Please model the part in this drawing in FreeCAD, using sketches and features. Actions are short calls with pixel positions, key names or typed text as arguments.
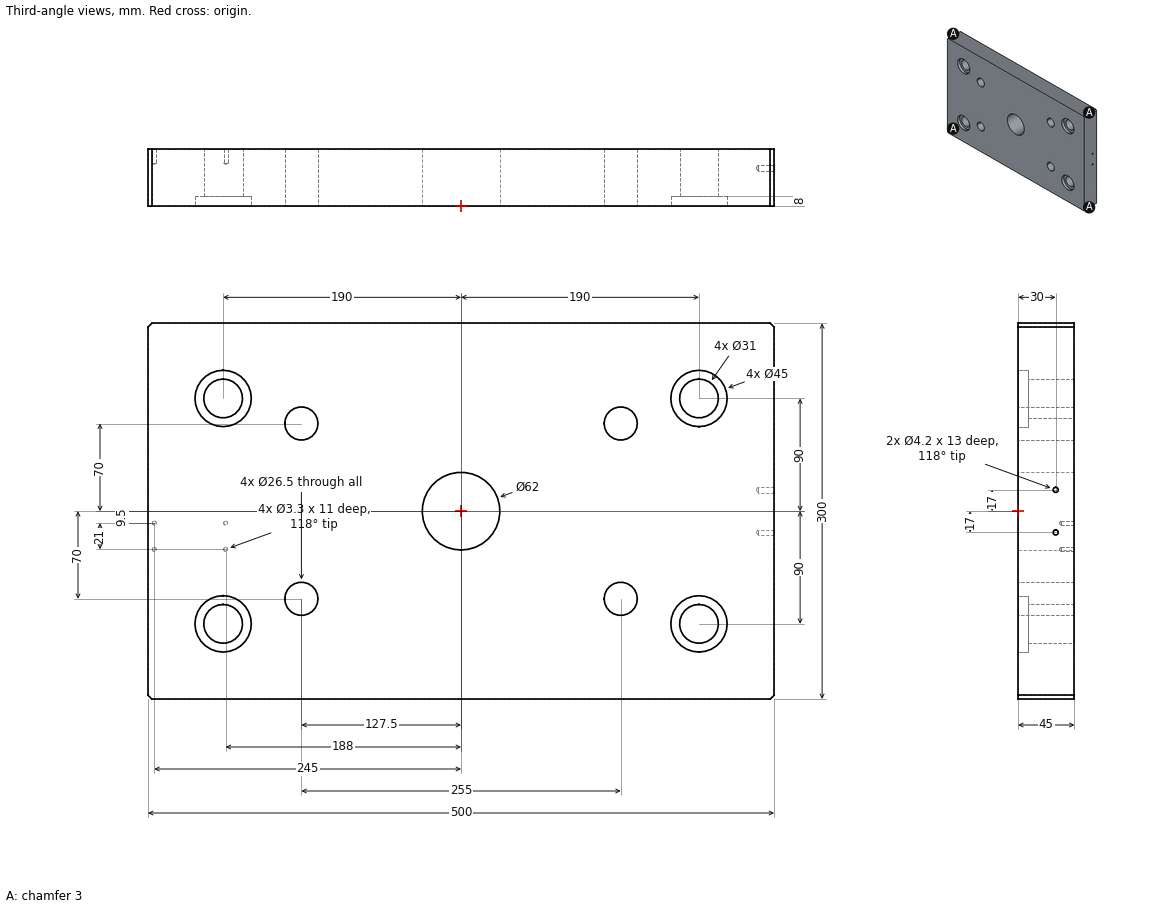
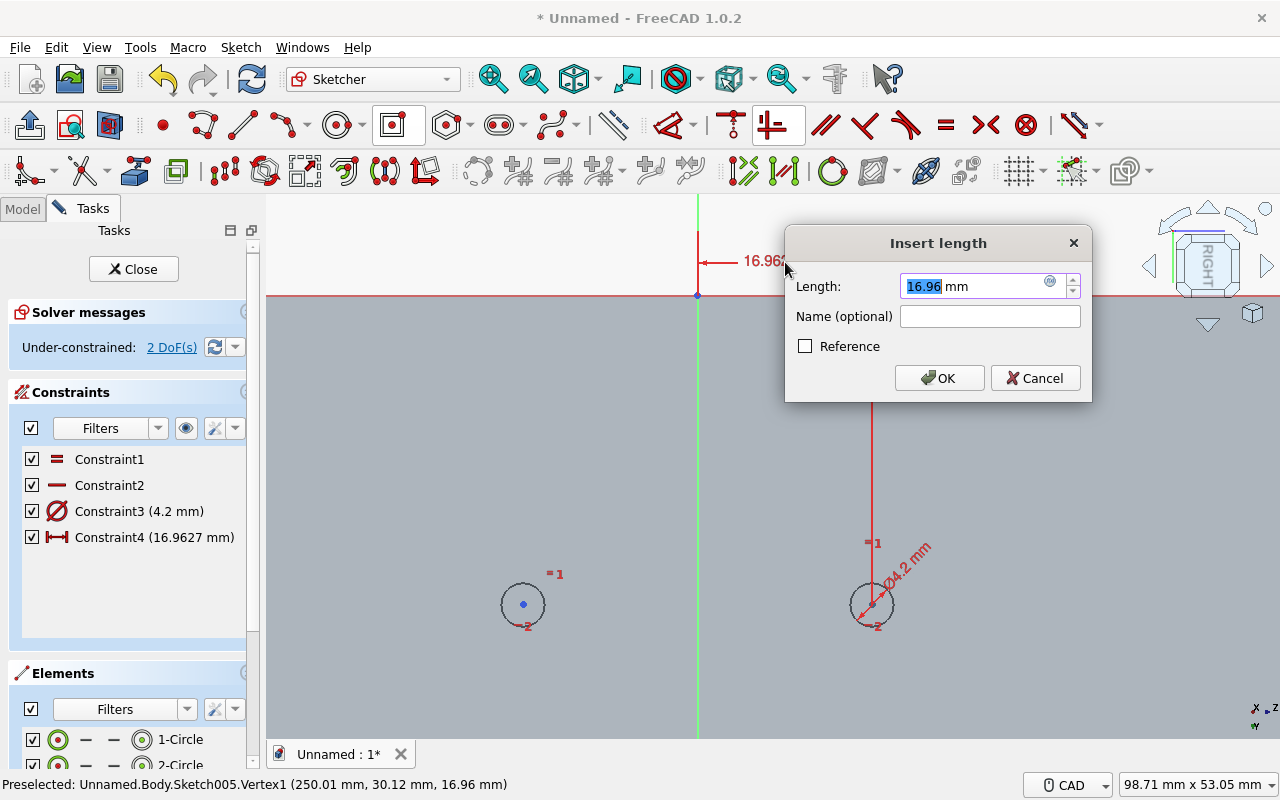
text(17)
key(Return)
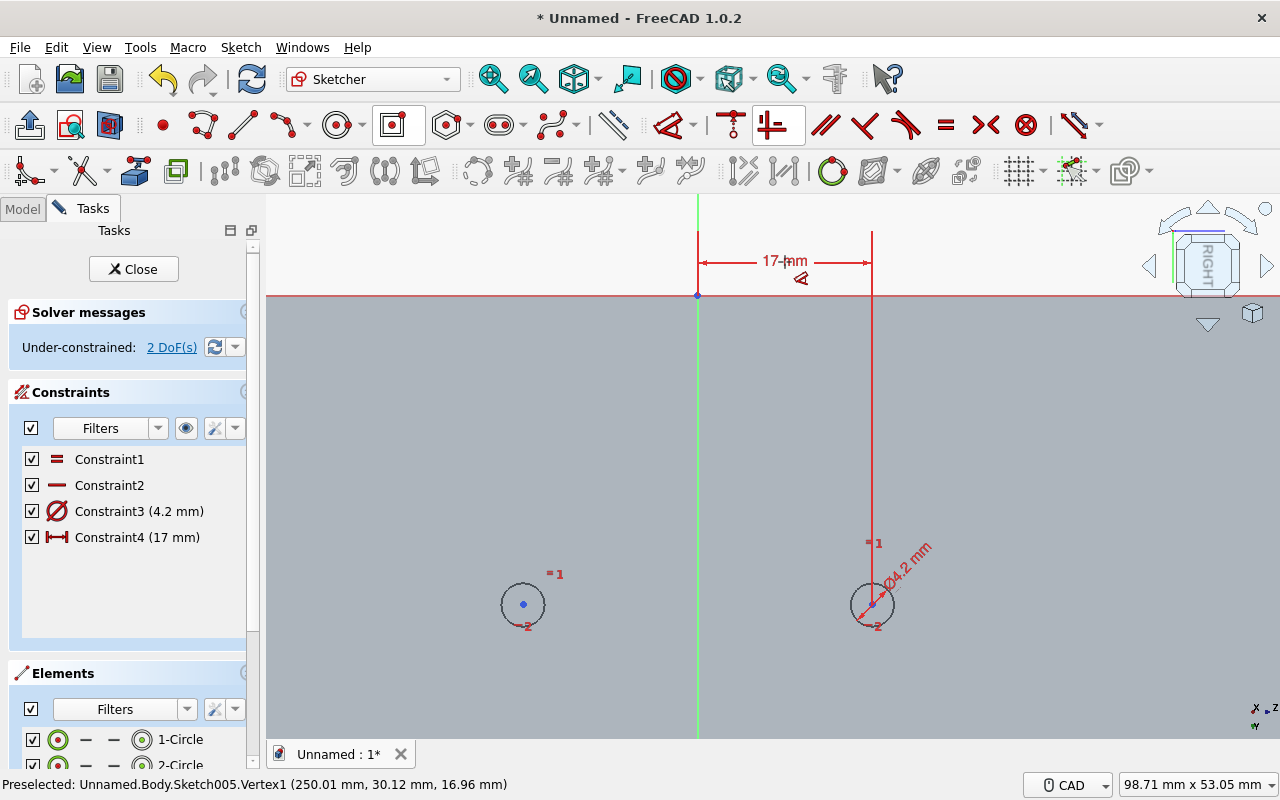
click(872, 605)
click(906, 450)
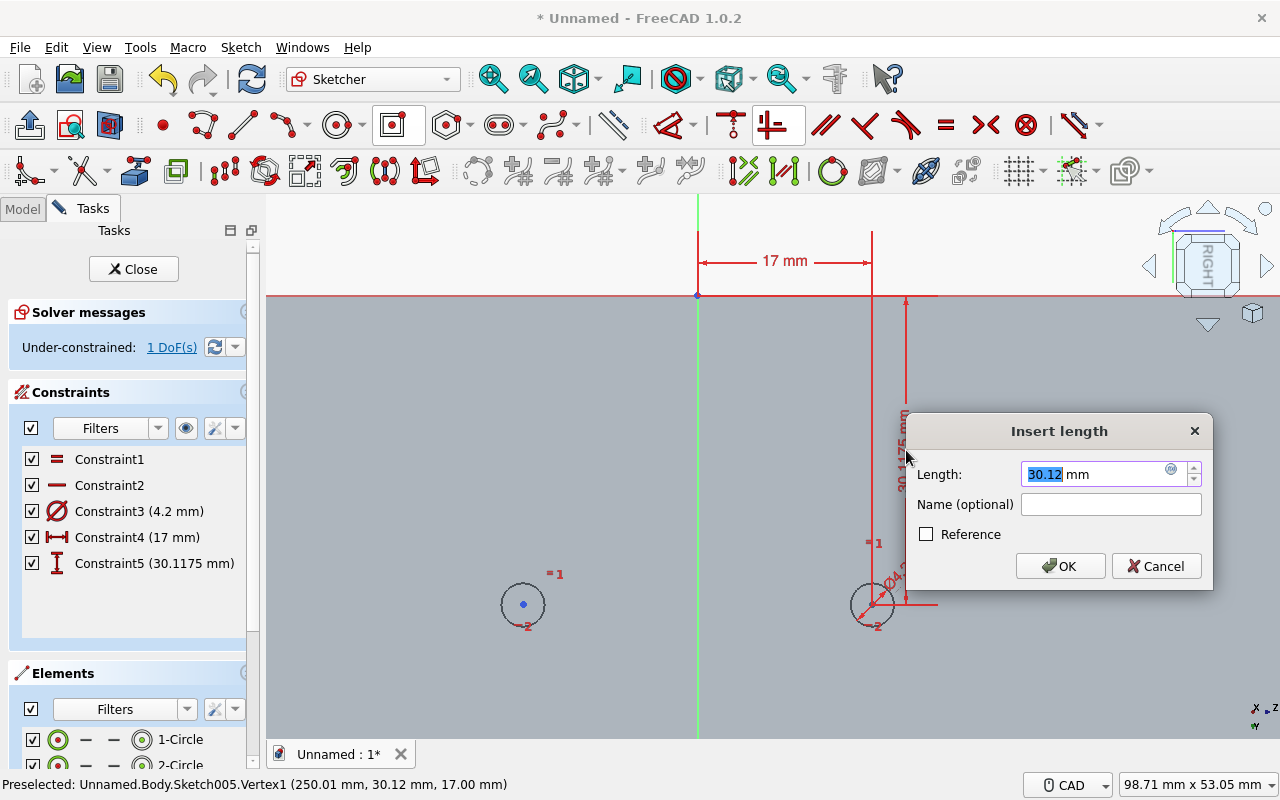
text(30)
key(Return)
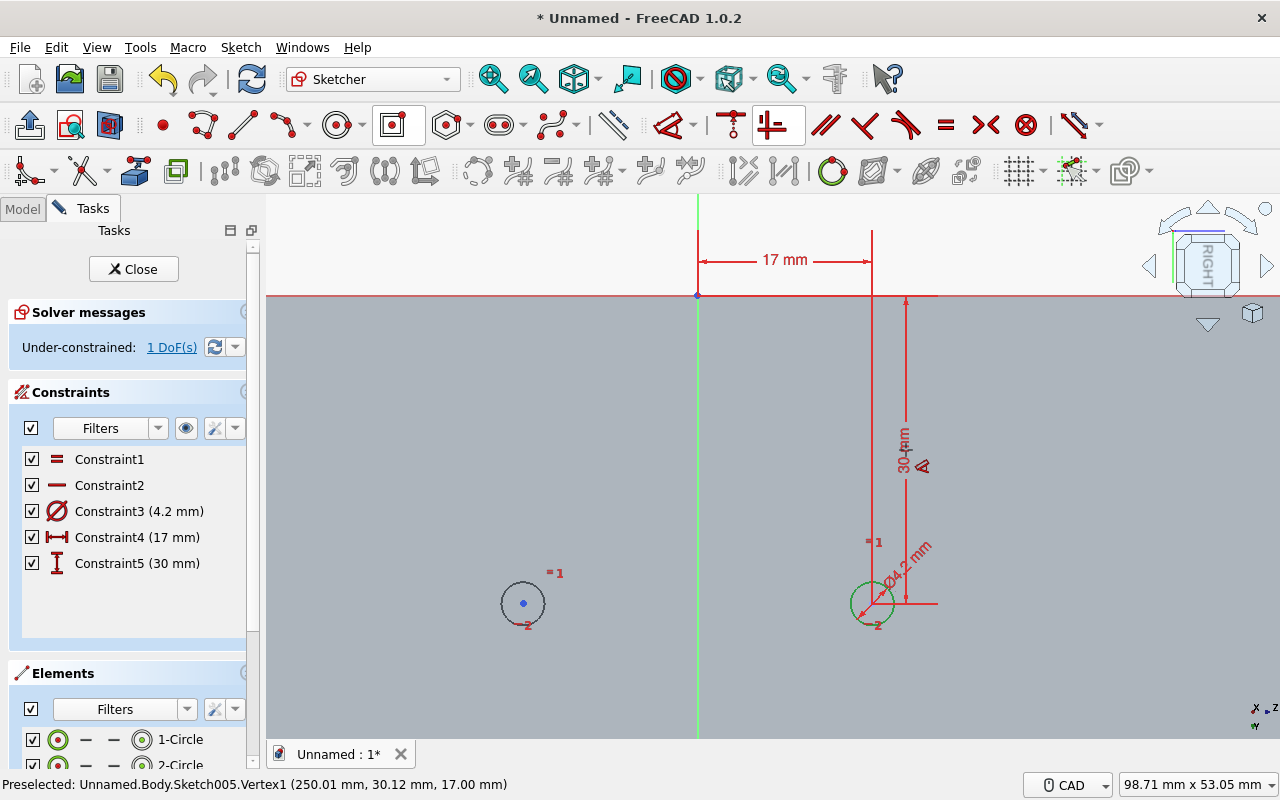
click(523, 604)
click(610, 262)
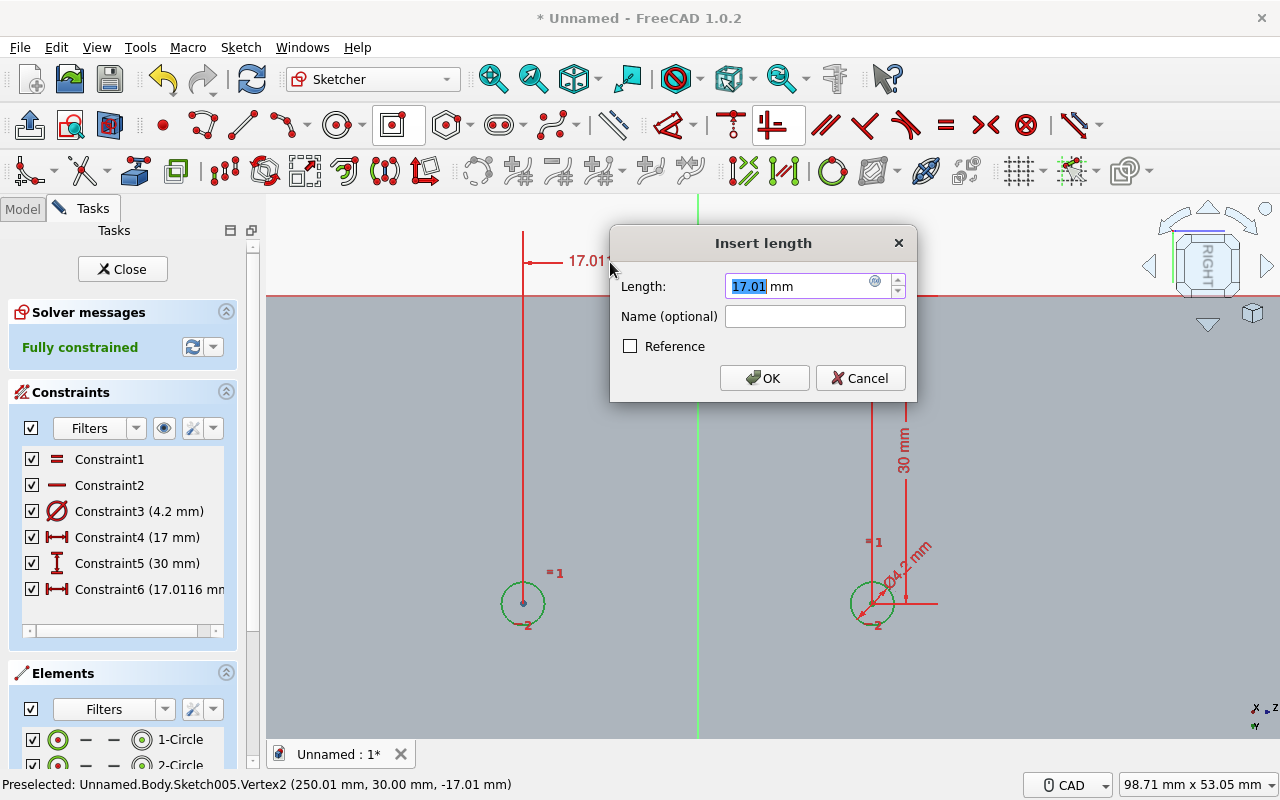
text(17)
key(Return)
key(Escape)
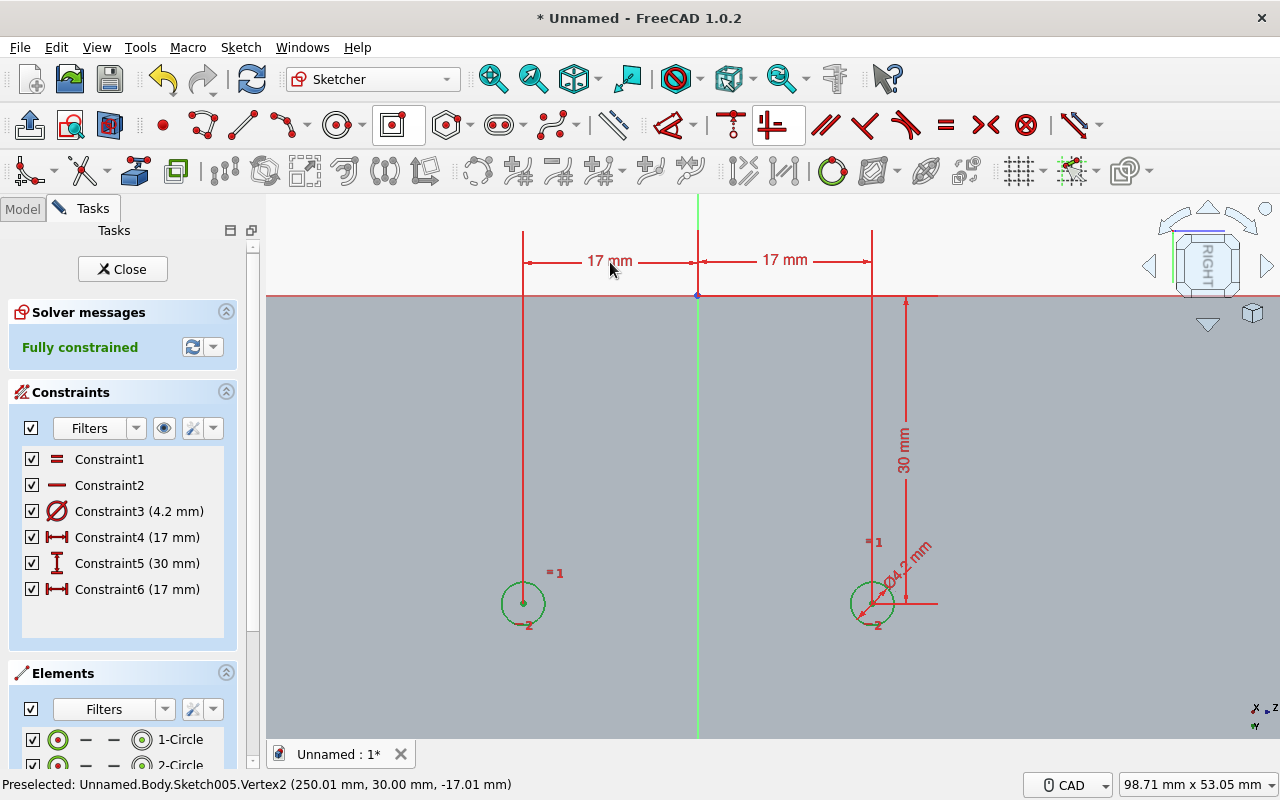
click(123, 269)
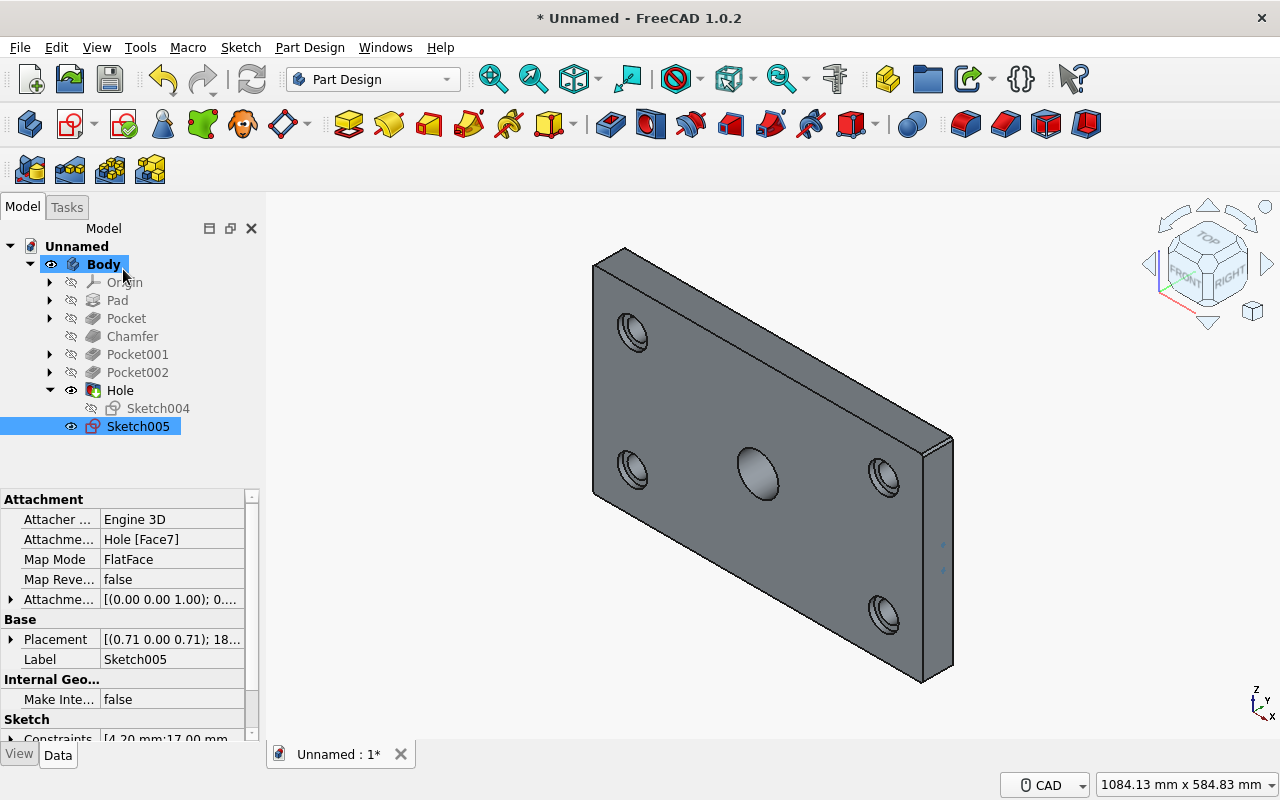
click(652, 124)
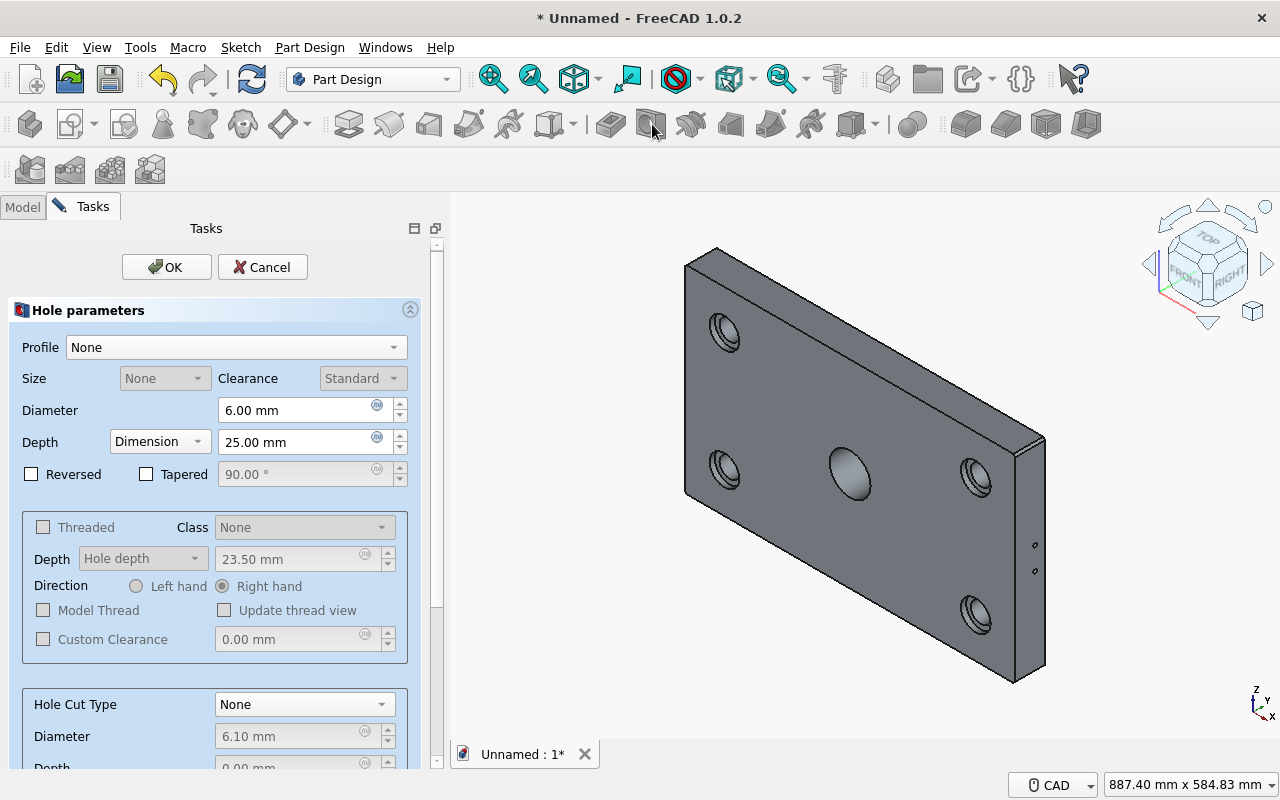
triple_click(305, 410)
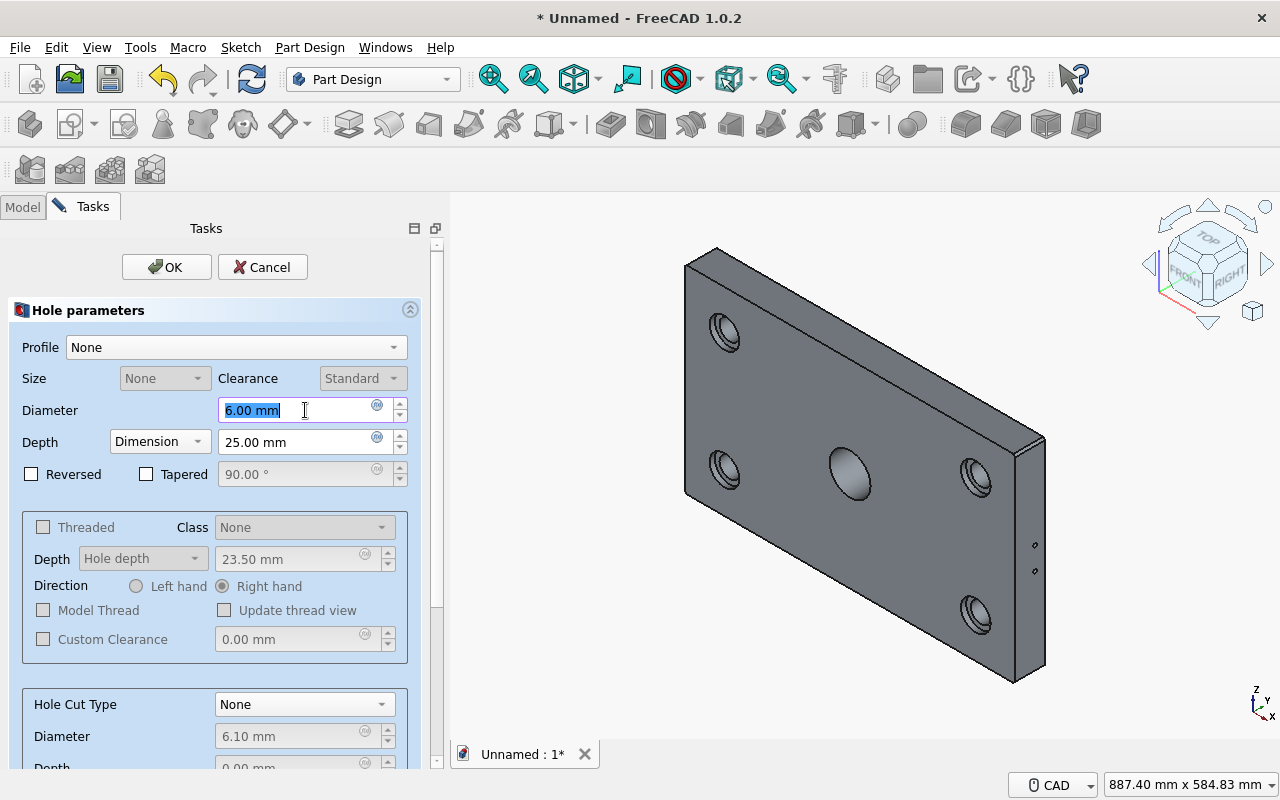
text(4.2)
key(Tab)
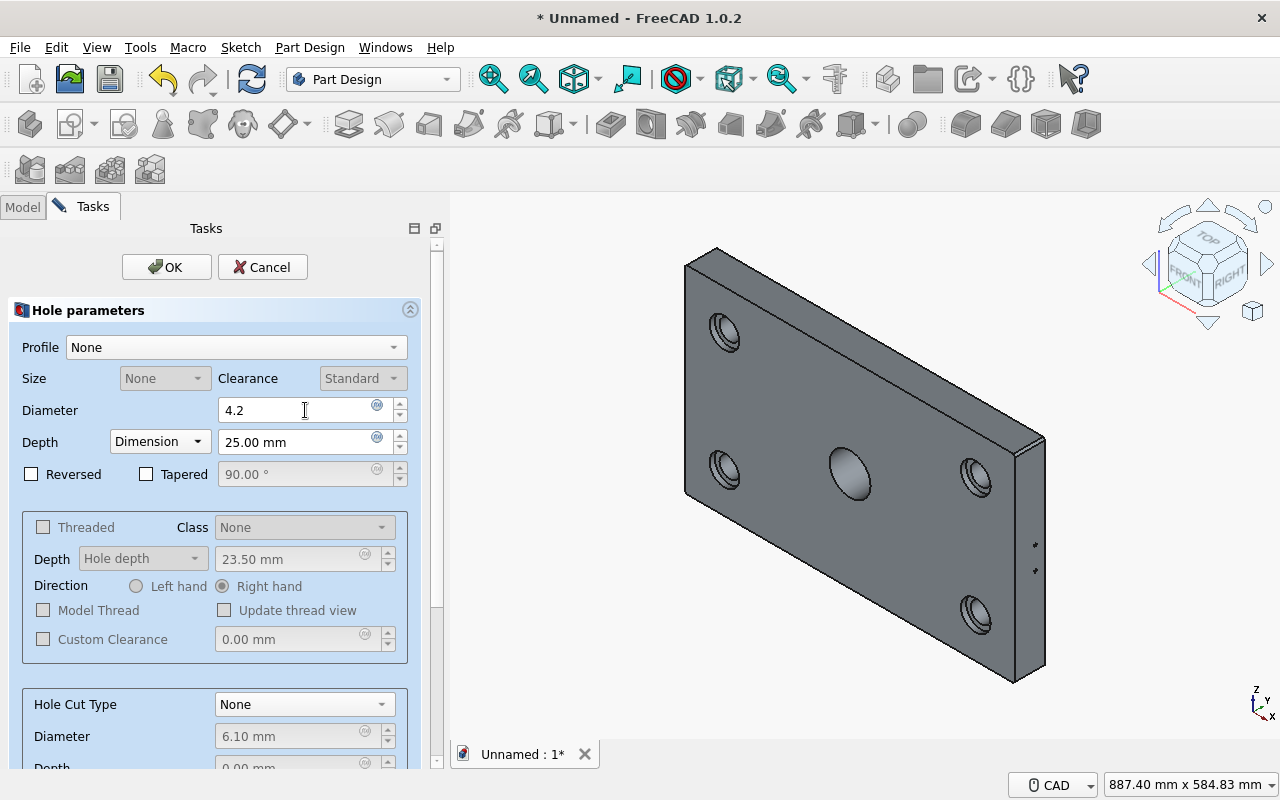
triple_click(305, 442)